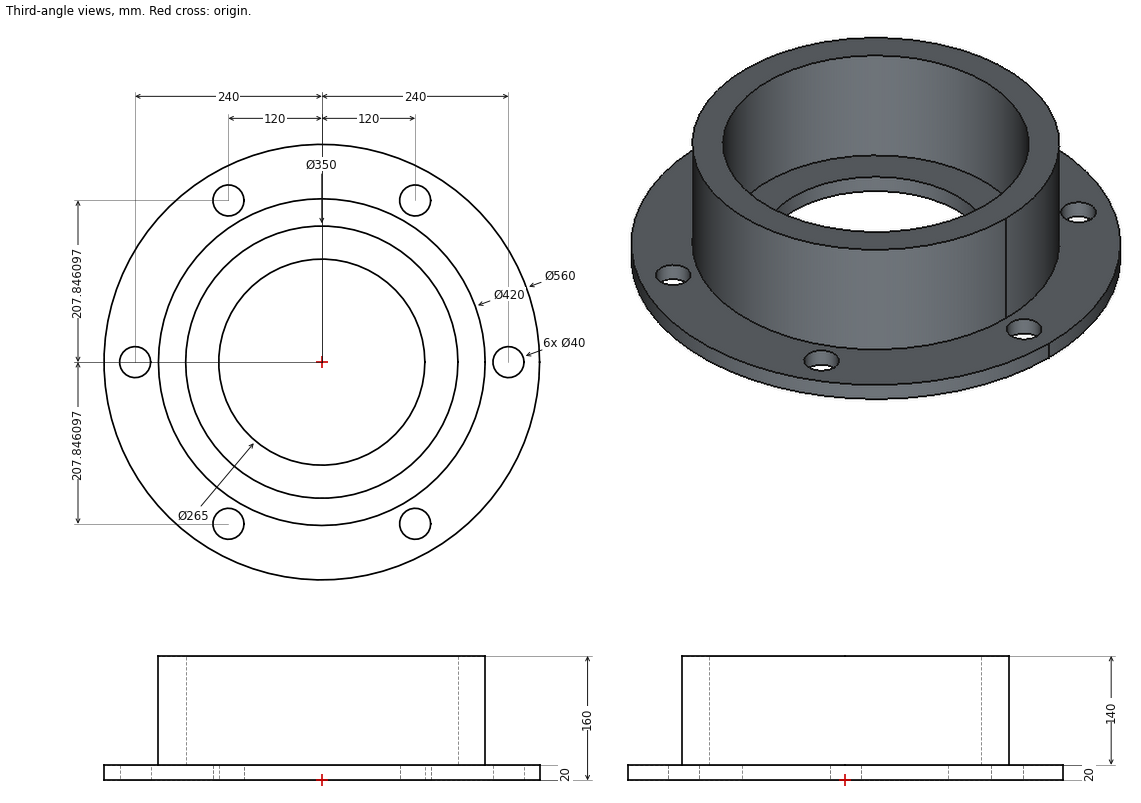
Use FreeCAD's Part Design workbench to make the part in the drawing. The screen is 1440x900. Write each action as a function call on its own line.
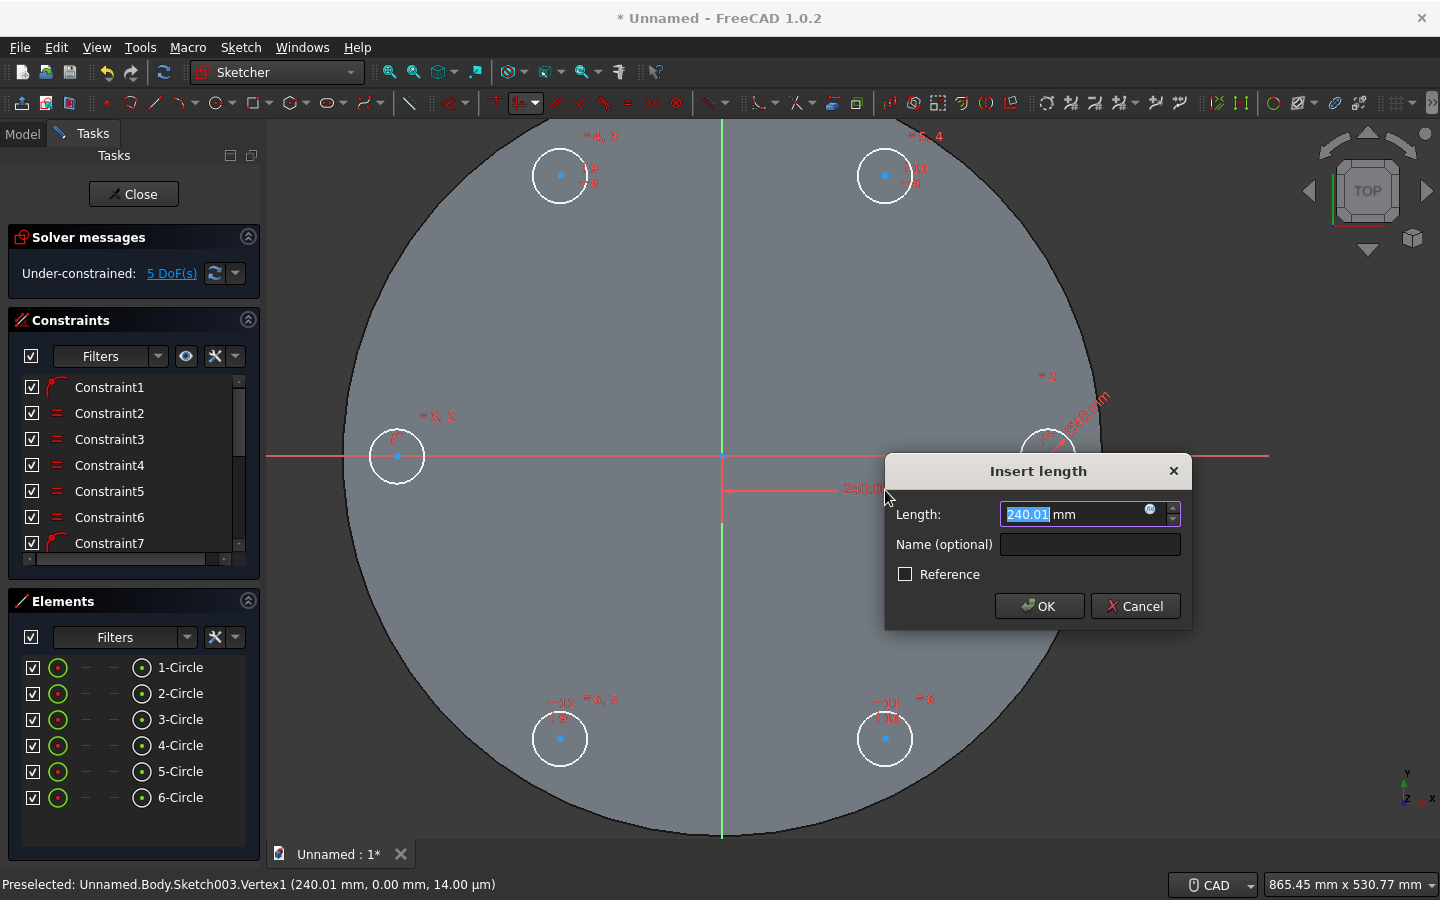
text(240)
key(Return)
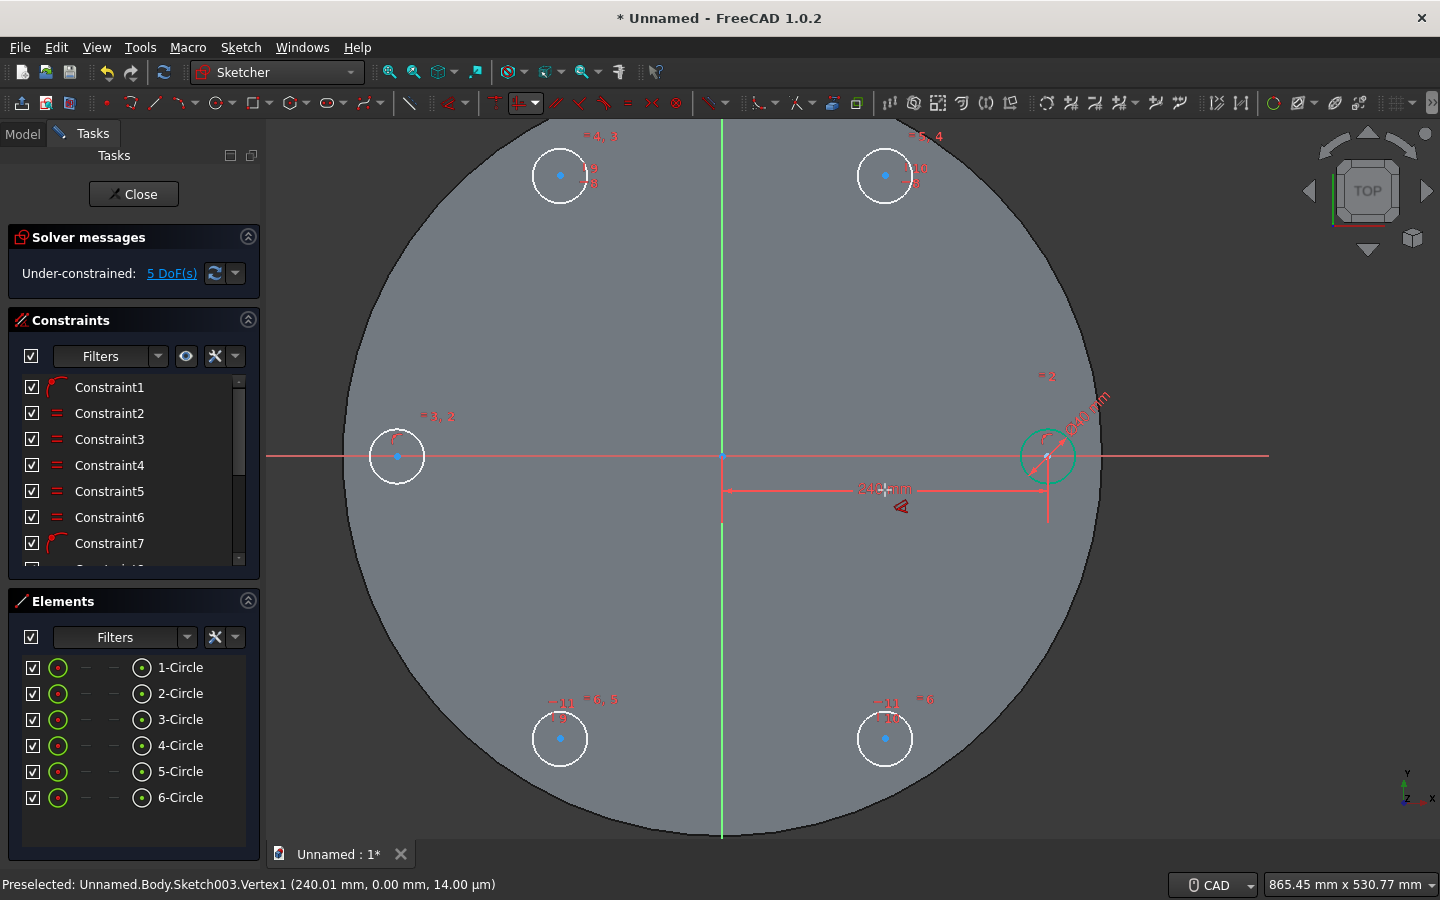
click(397, 456)
click(560, 490)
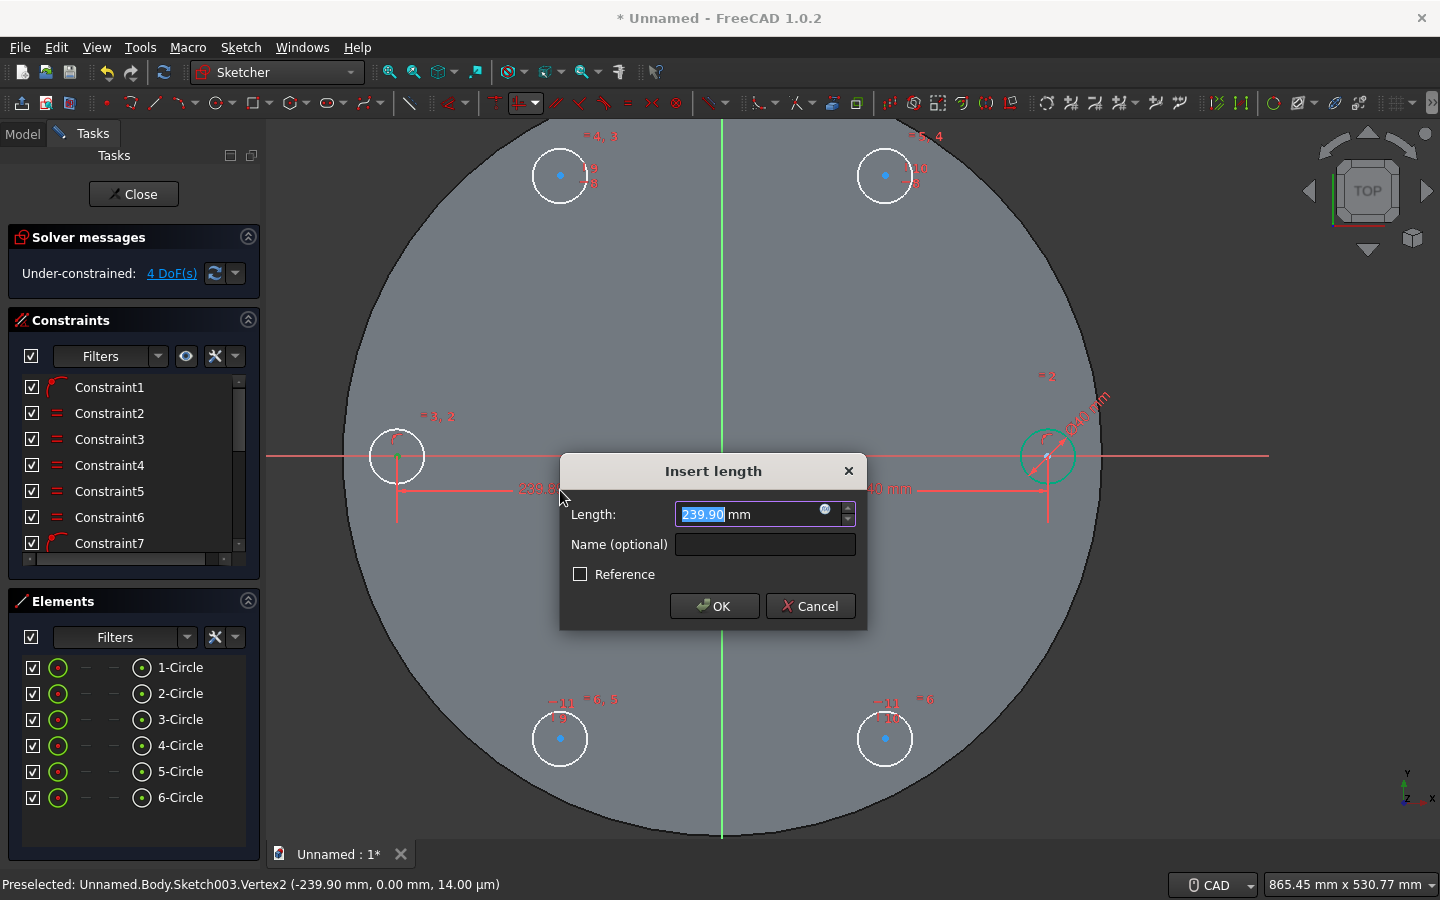
text(240)
key(Return)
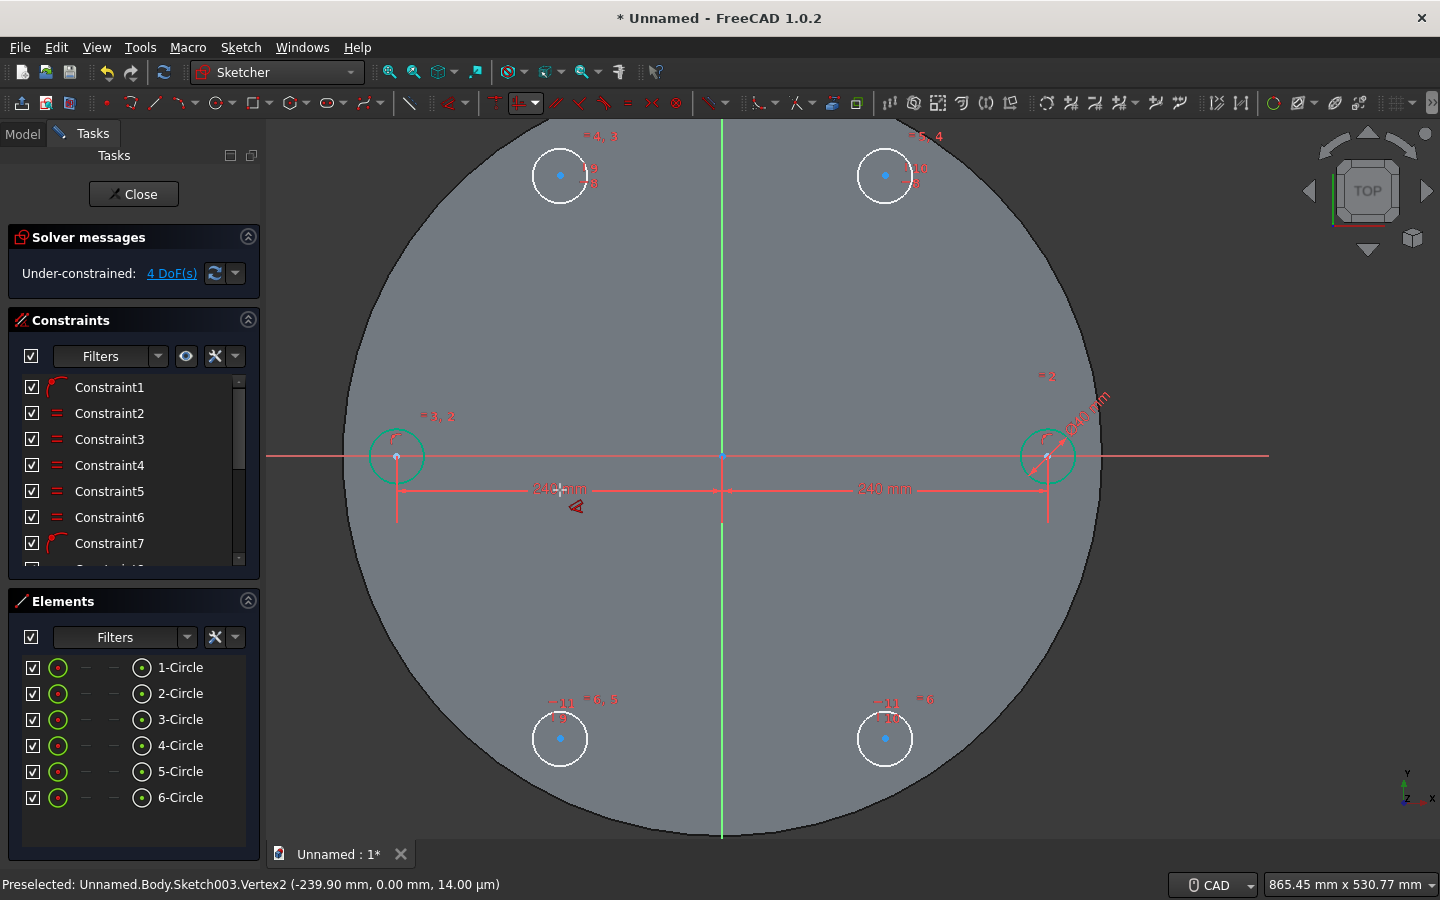
click(560, 176)
click(641, 490)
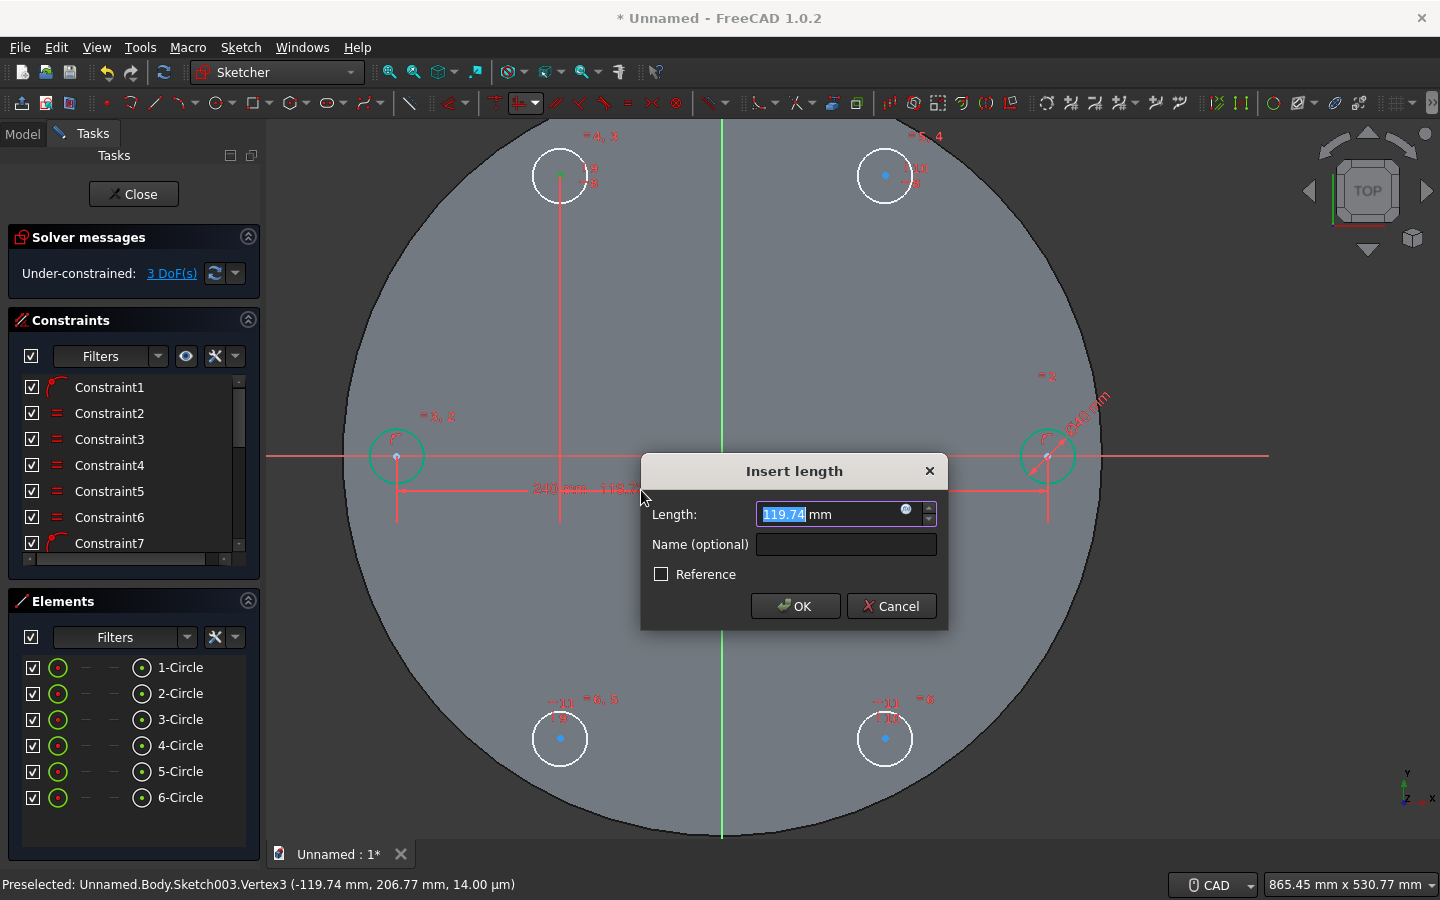
text(120)
key(Return)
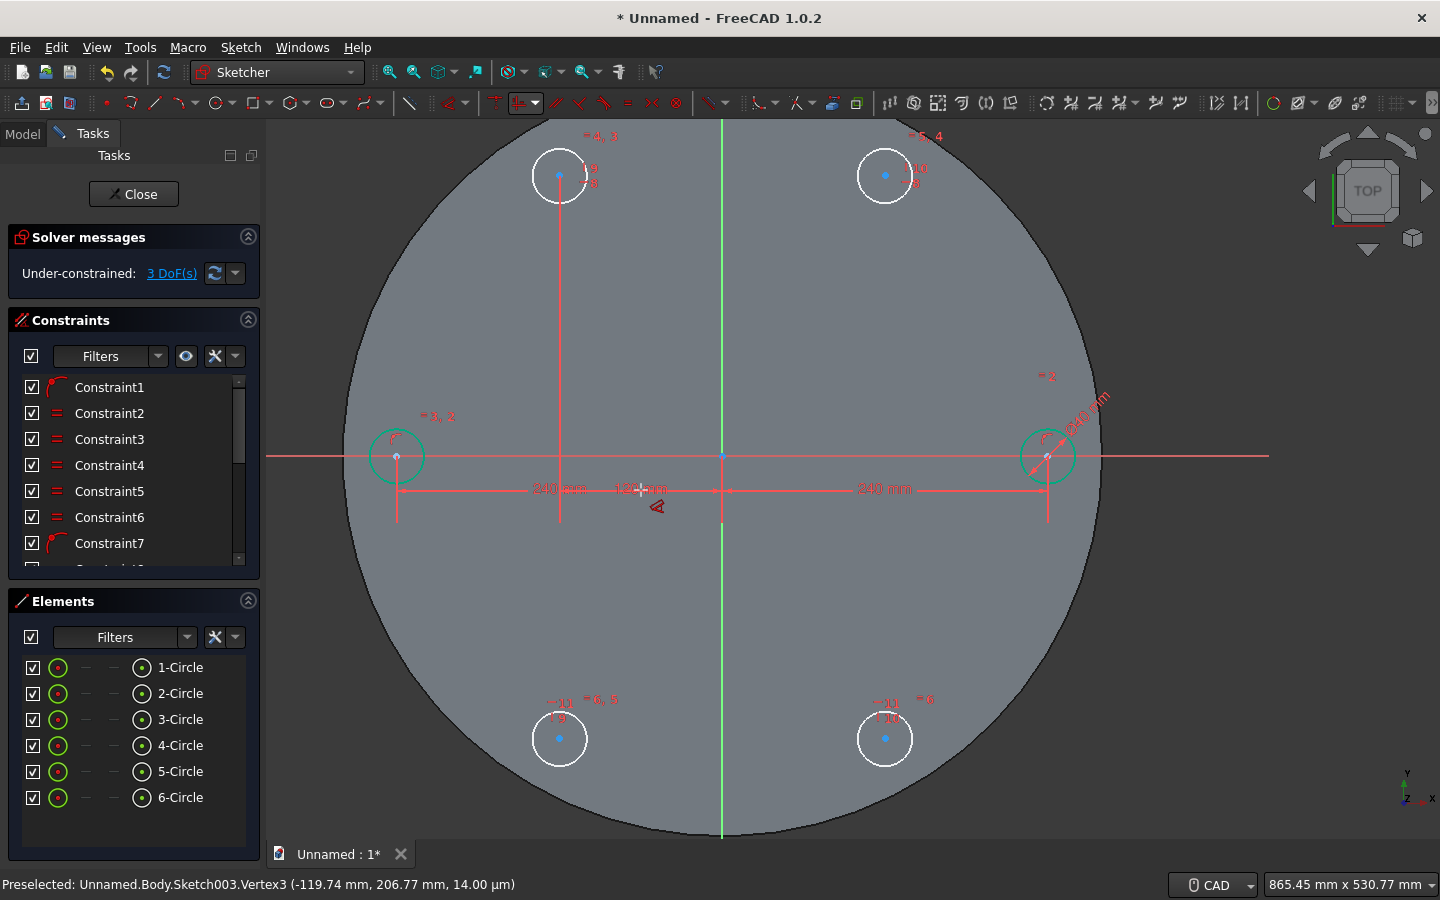
click(885, 176)
click(804, 490)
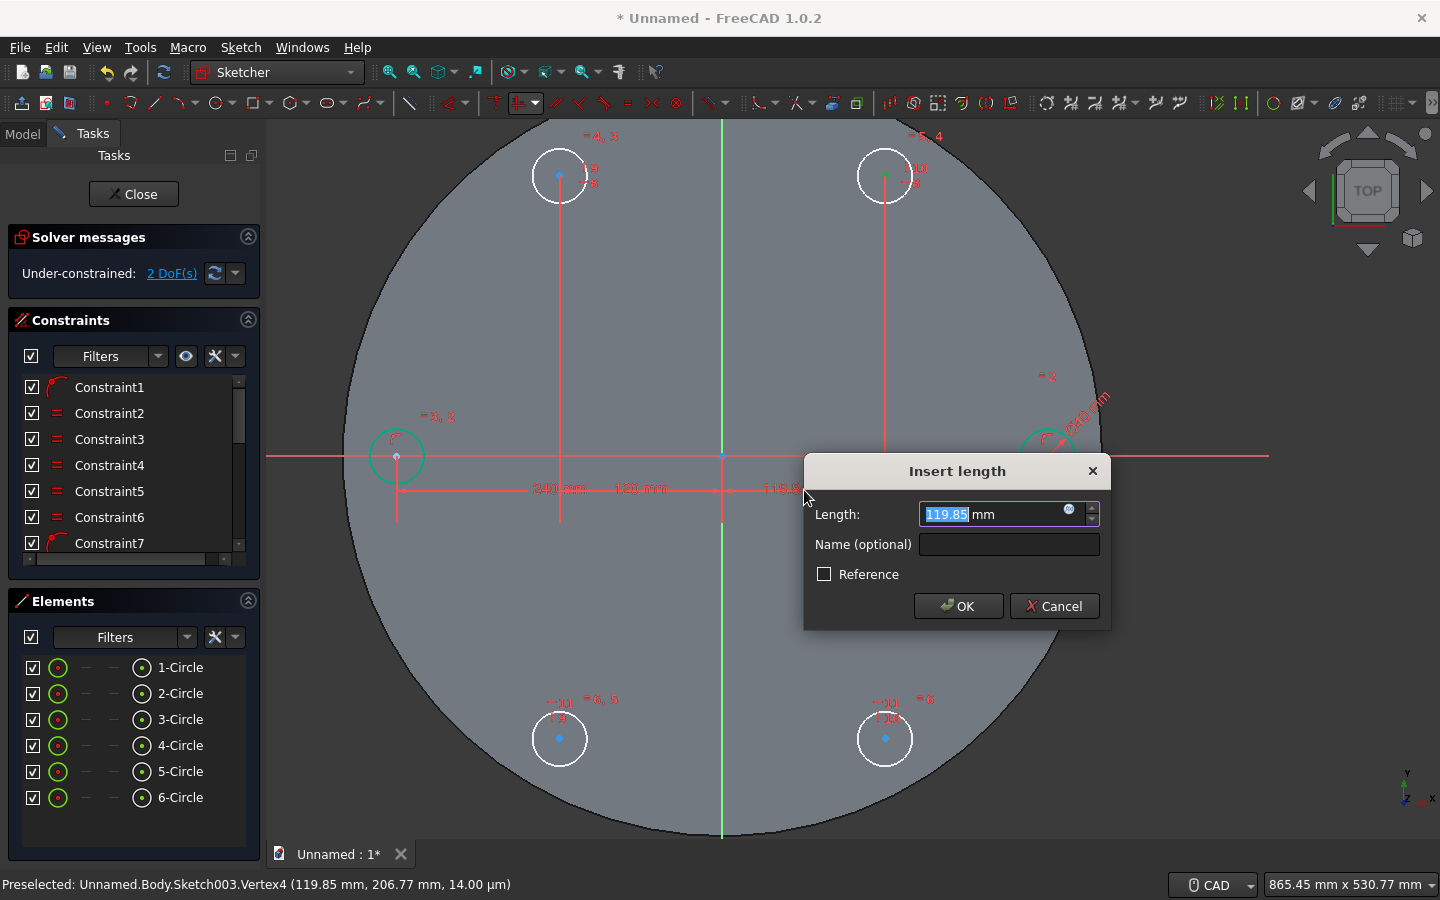
text(120)
key(Return)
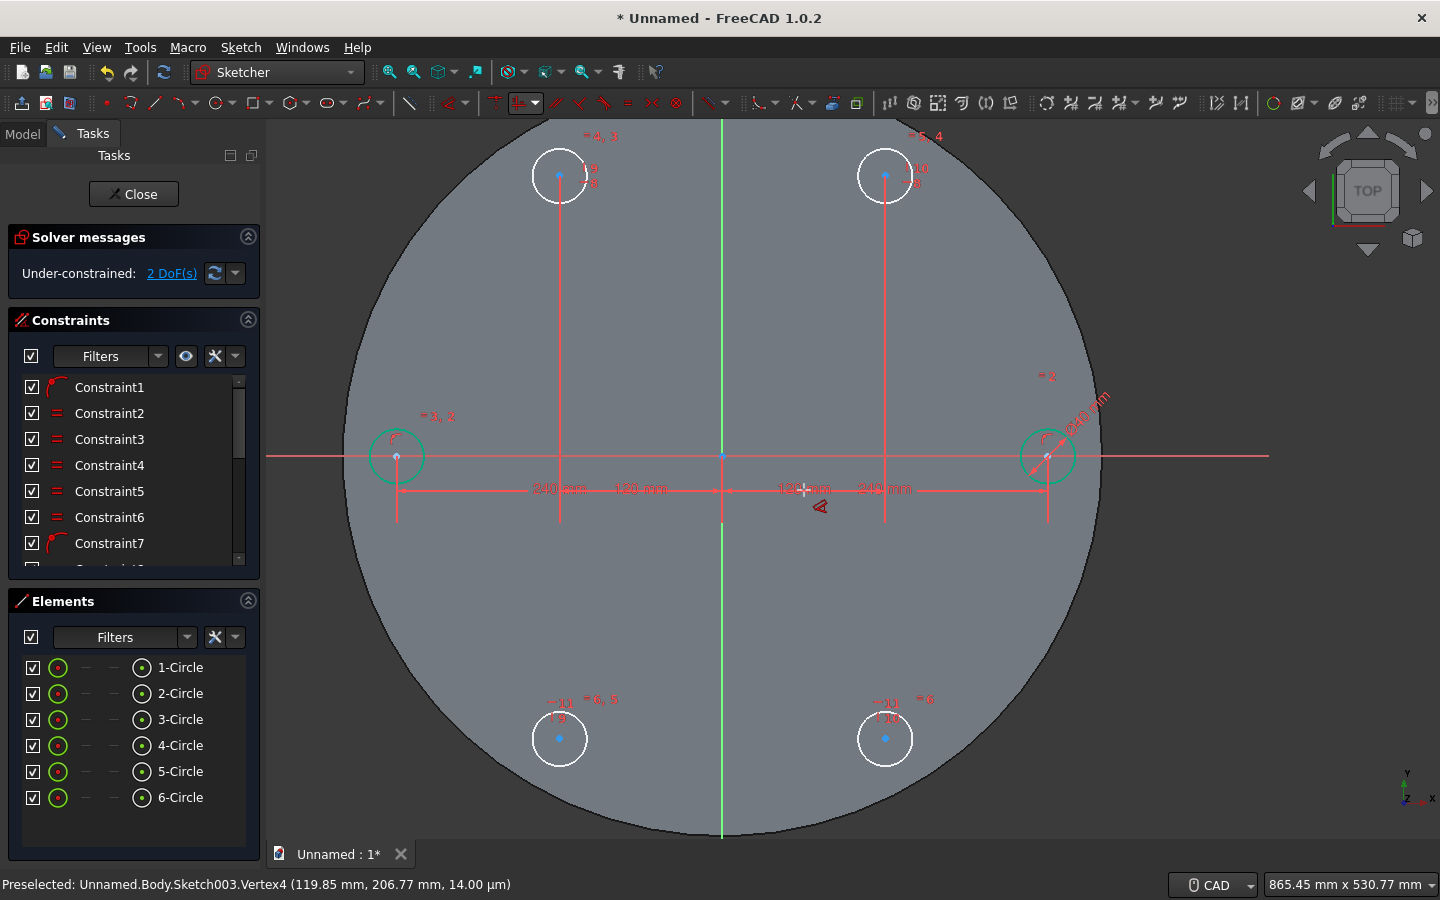
click(560, 176)
click(526, 316)